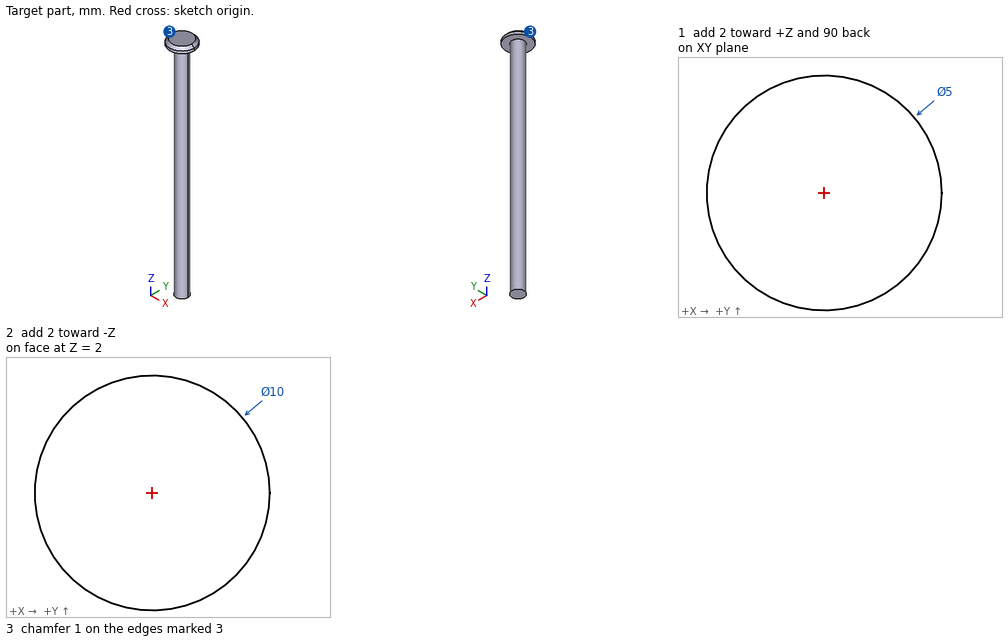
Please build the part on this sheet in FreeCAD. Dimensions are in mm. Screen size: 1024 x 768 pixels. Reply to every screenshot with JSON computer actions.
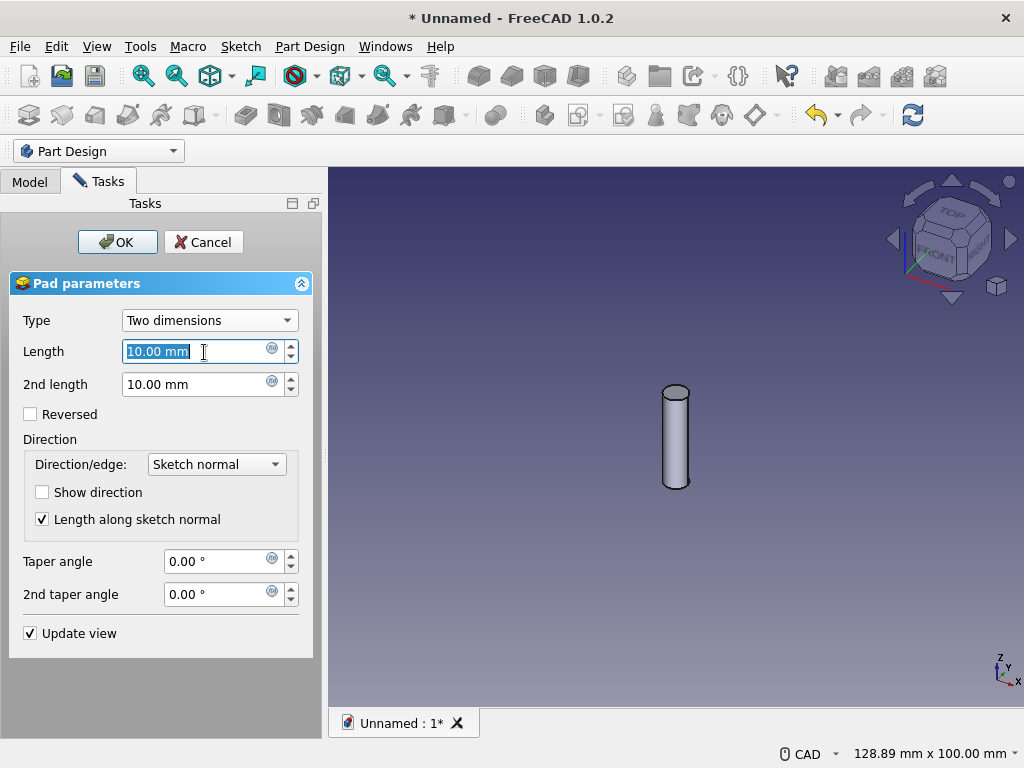
{"action": "type", "text": "2"}
{"action": "key", "text": "Tab"}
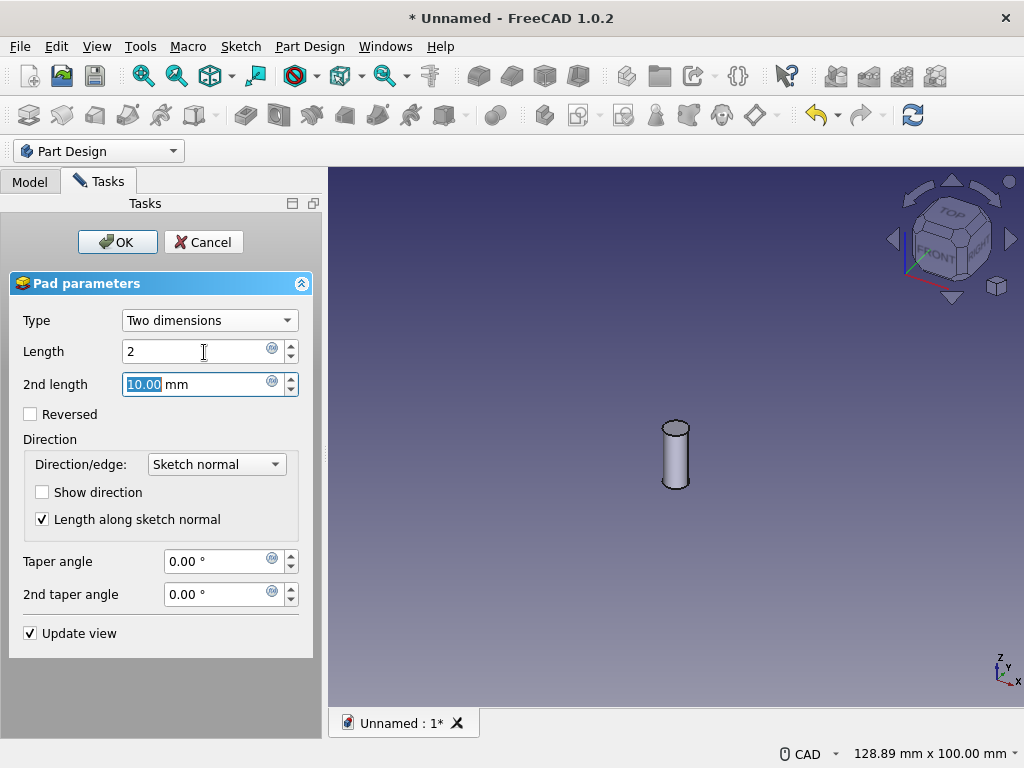
{"action": "type", "text": "90"}
{"action": "key", "text": "Tab"}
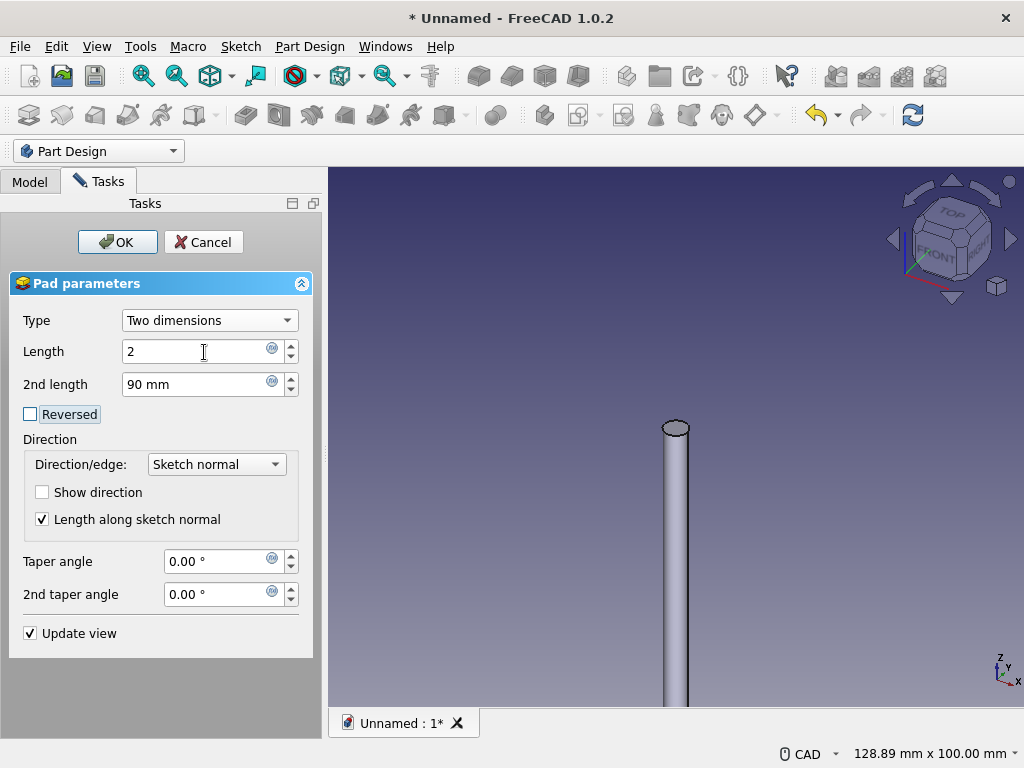
{"action": "left_click", "coordinate": [118, 242]}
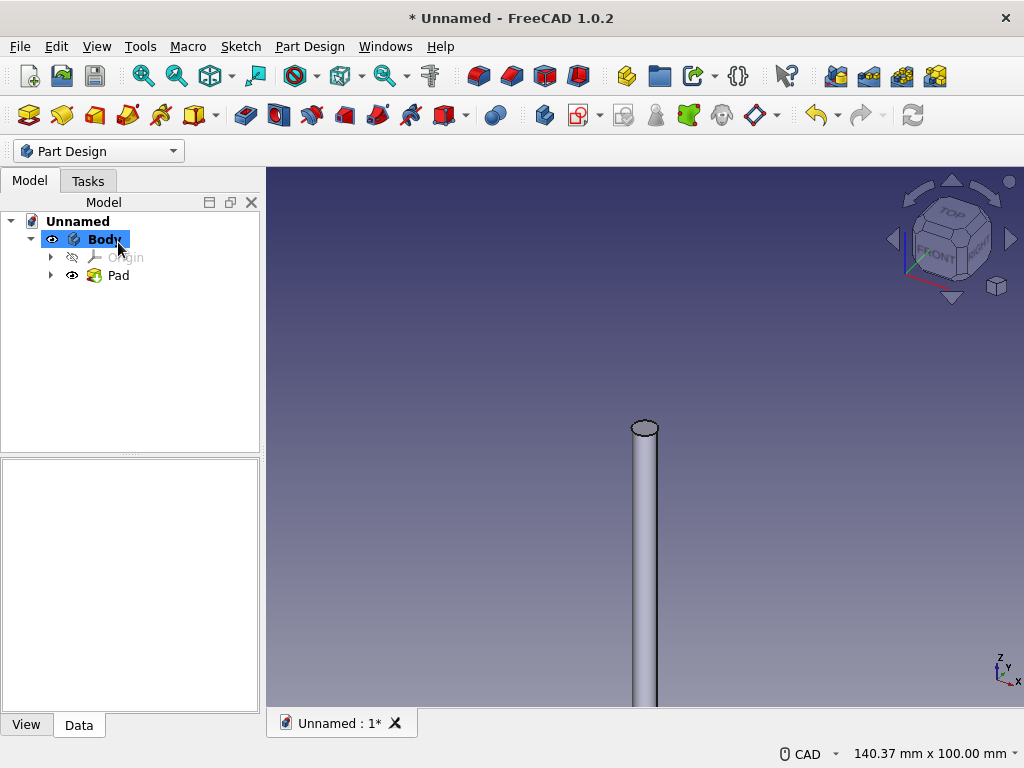
{"action": "key", "text": "v f"}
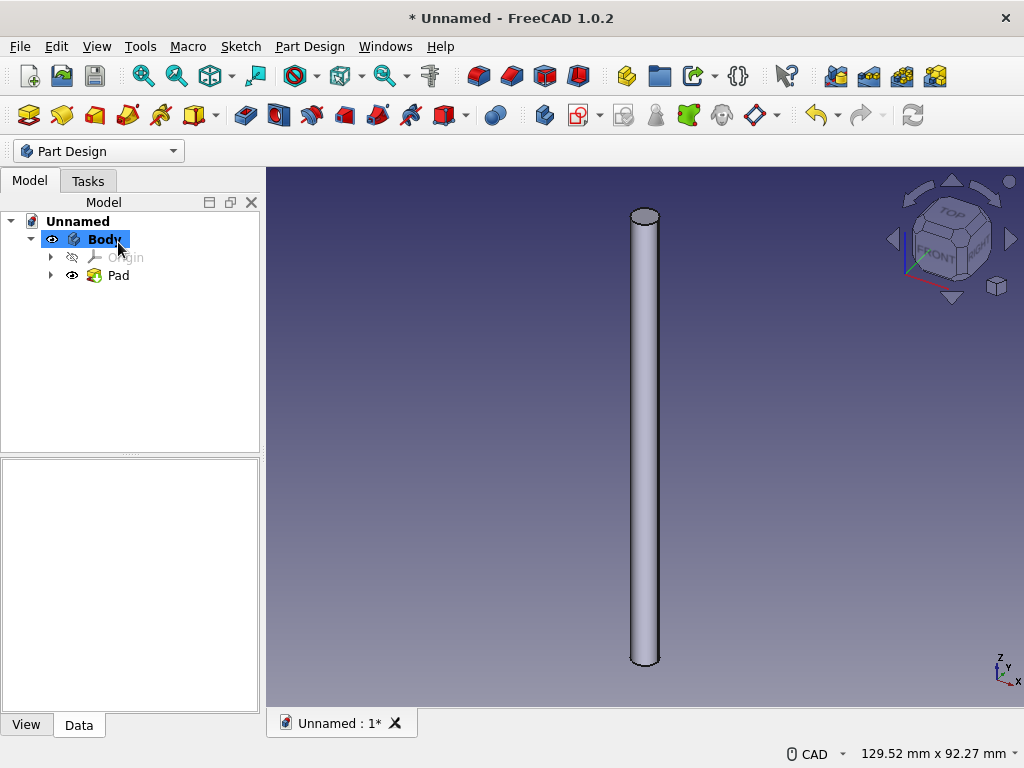
{"action": "left_click", "coordinate": [645, 215]}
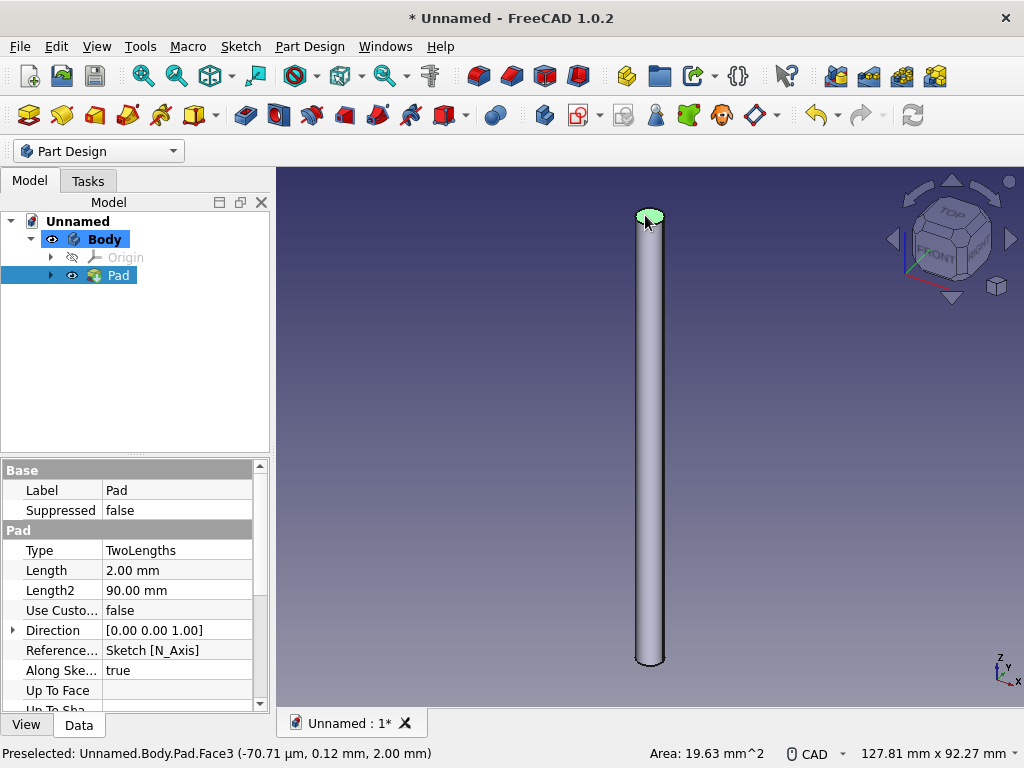
{"action": "left_click", "coordinate": [578, 116]}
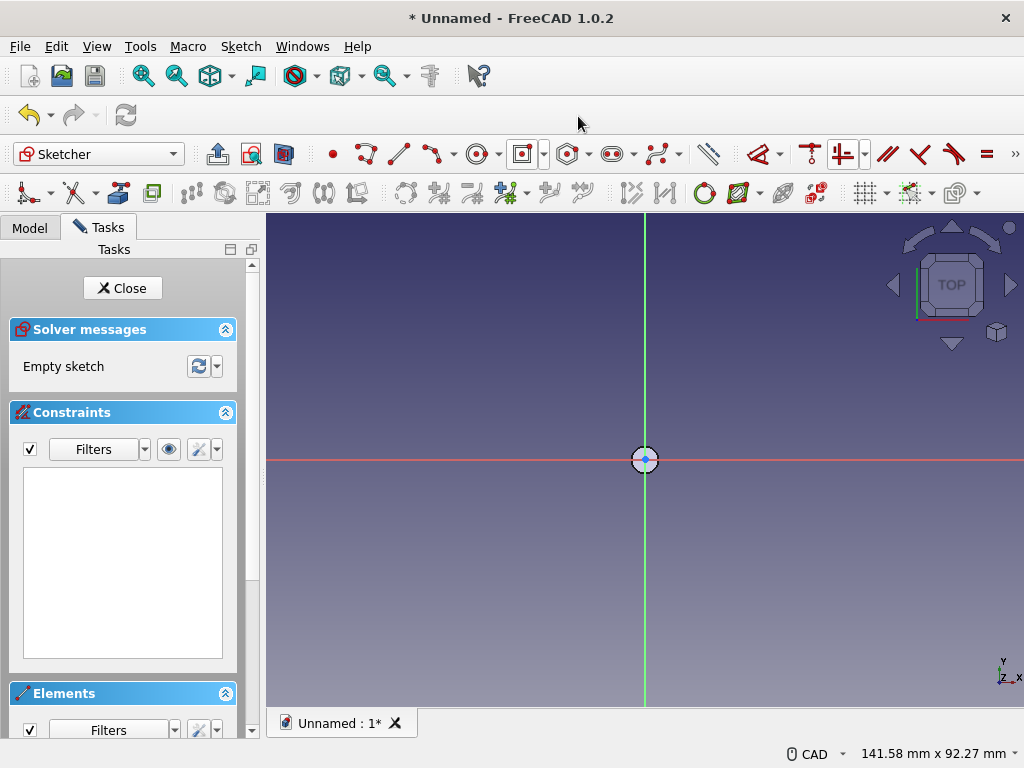
{"action": "scroll", "coordinate": [659, 460], "scroll_direction": "up", "scroll_amount": 9}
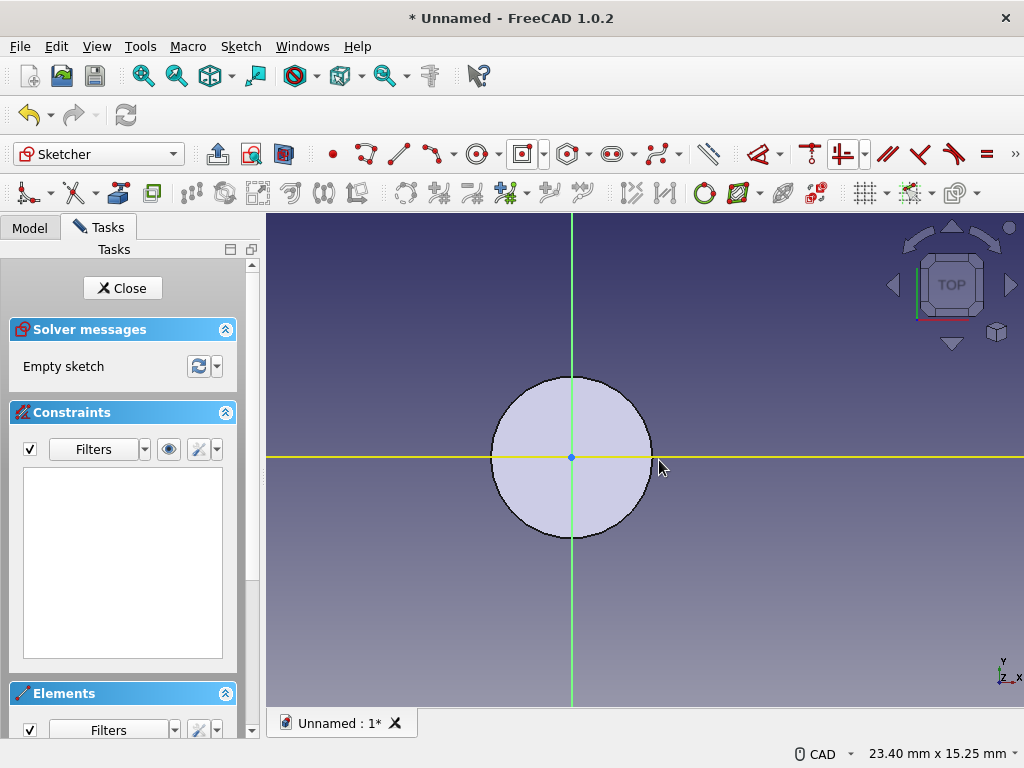
{"action": "key", "text": "g c"}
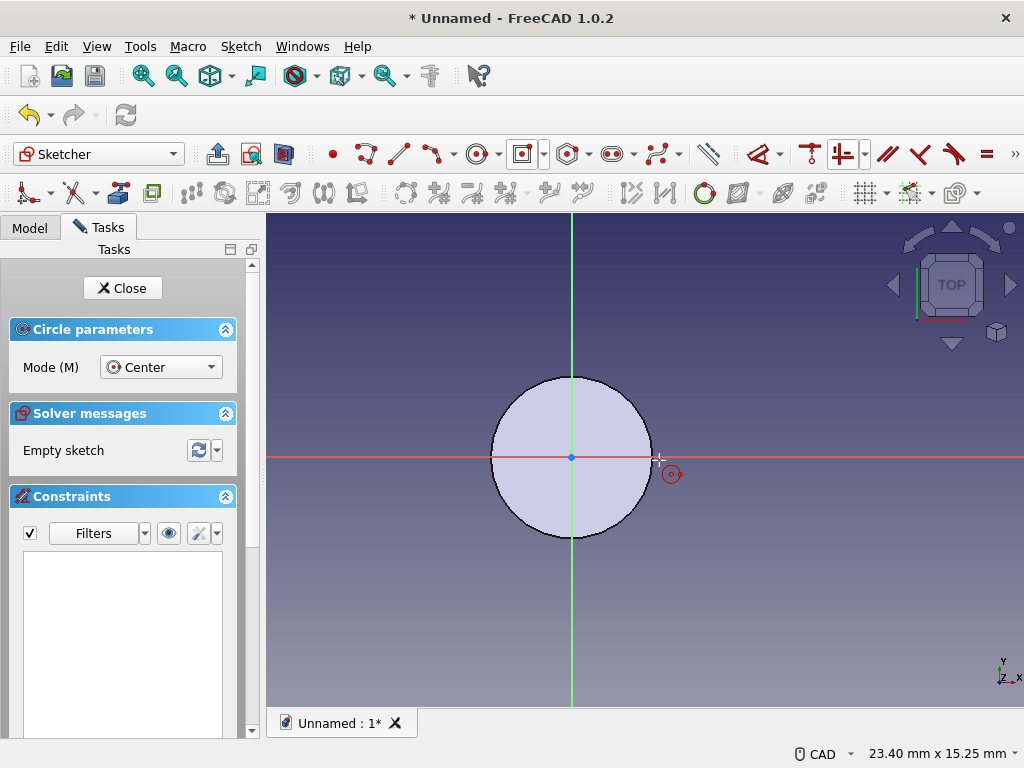
{"action": "left_click", "coordinate": [572, 457]}
{"action": "mouse_move", "coordinate": [686, 343]}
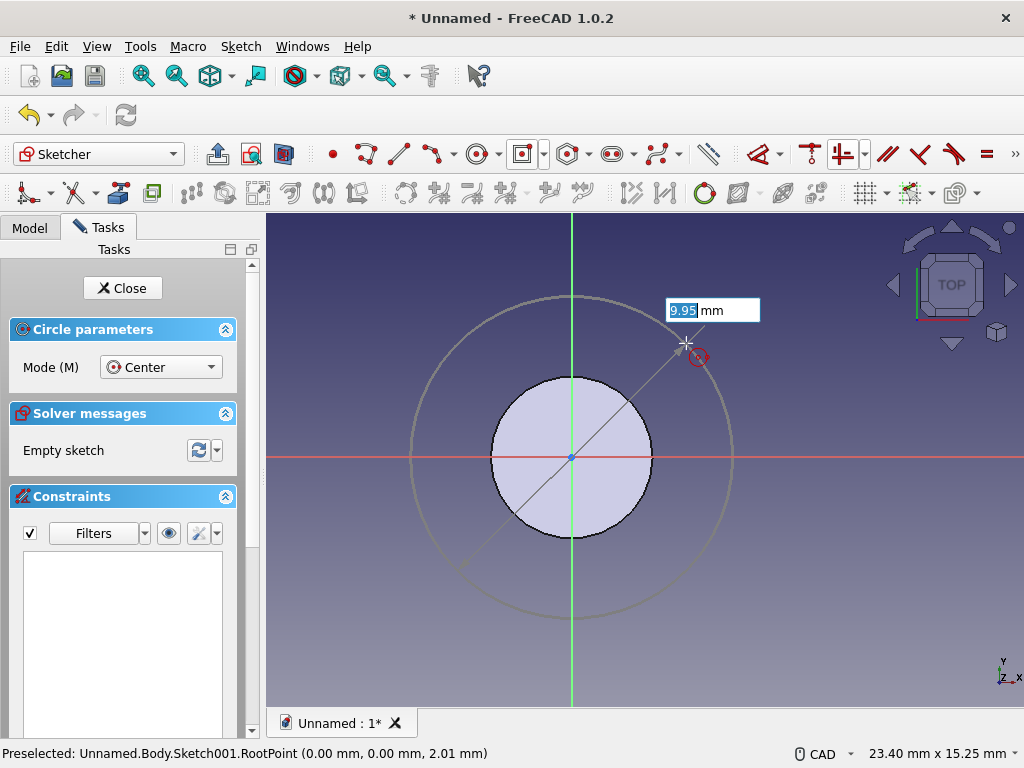
{"action": "type", "text": "10"}
{"action": "key", "text": "Return"}
{"action": "key", "text": "Escape"}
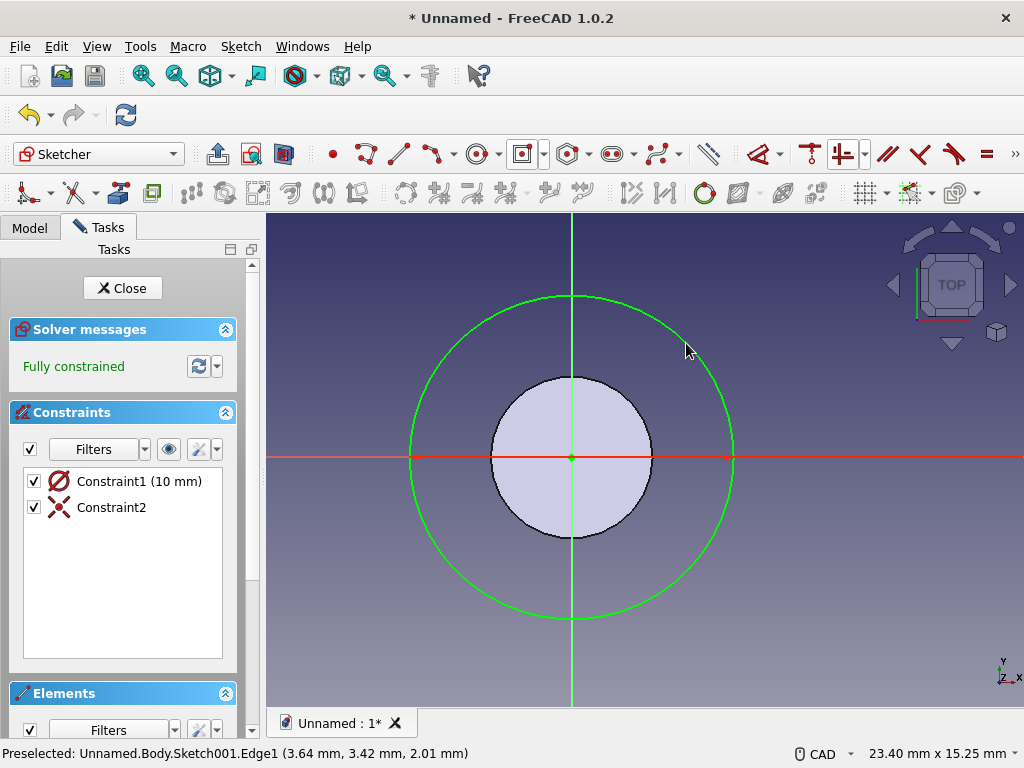
{"action": "left_click", "coordinate": [123, 288]}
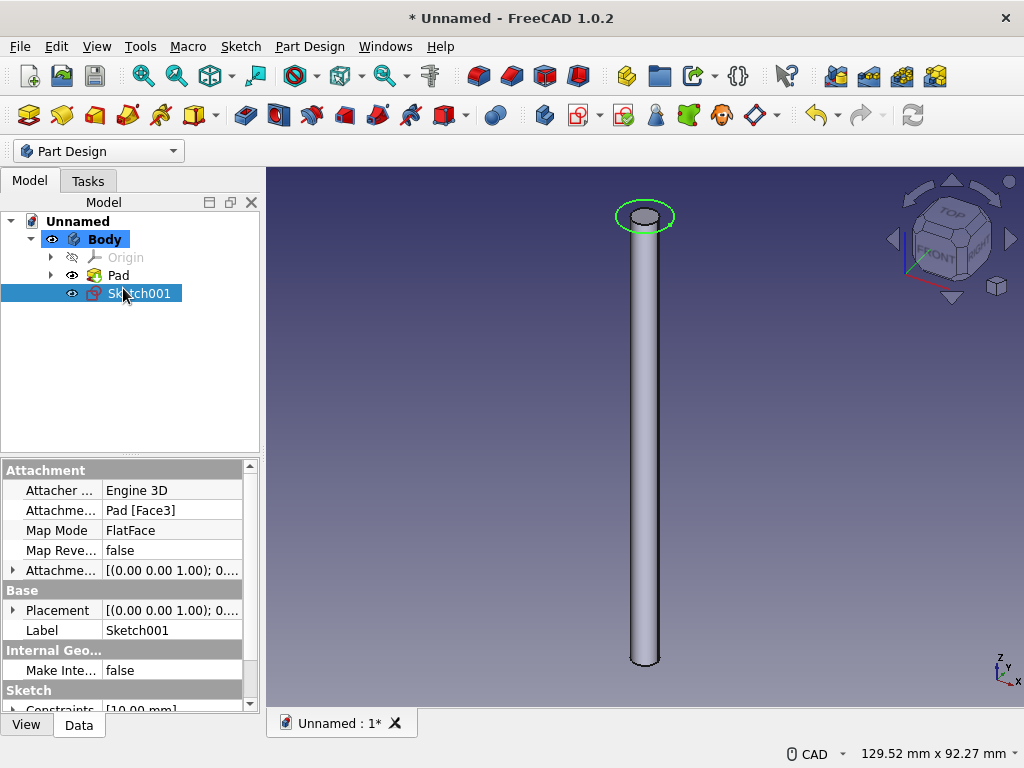
{"action": "left_click", "coordinate": [29, 116]}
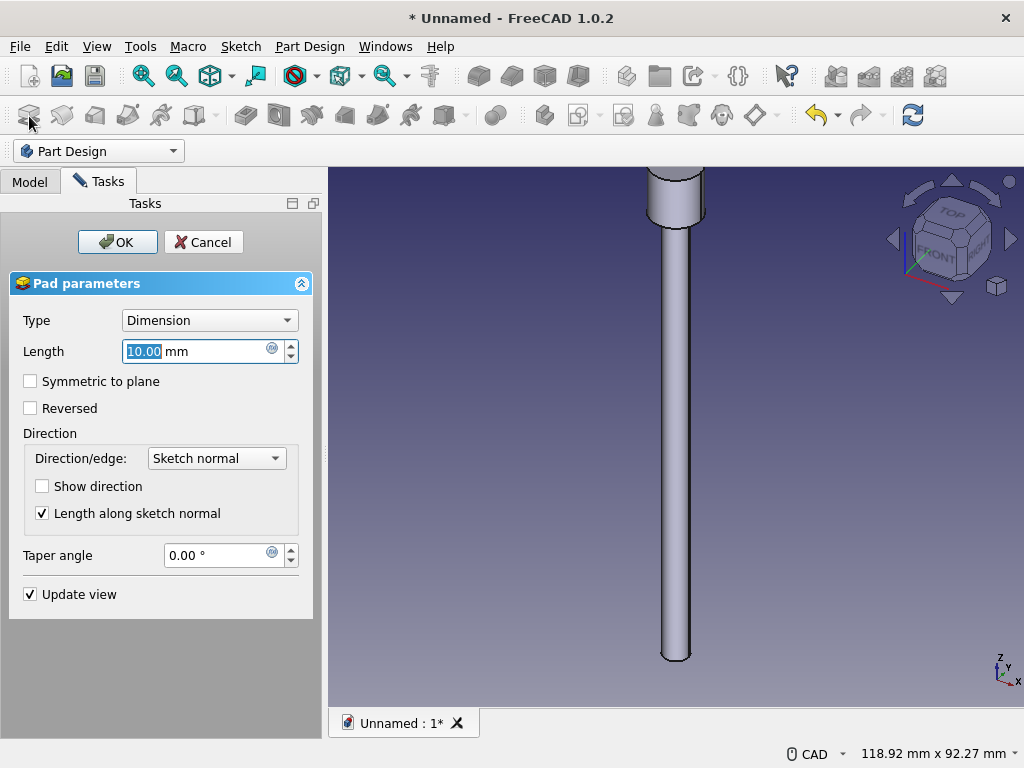
{"action": "type", "text": "2"}
{"action": "key", "text": "Tab"}